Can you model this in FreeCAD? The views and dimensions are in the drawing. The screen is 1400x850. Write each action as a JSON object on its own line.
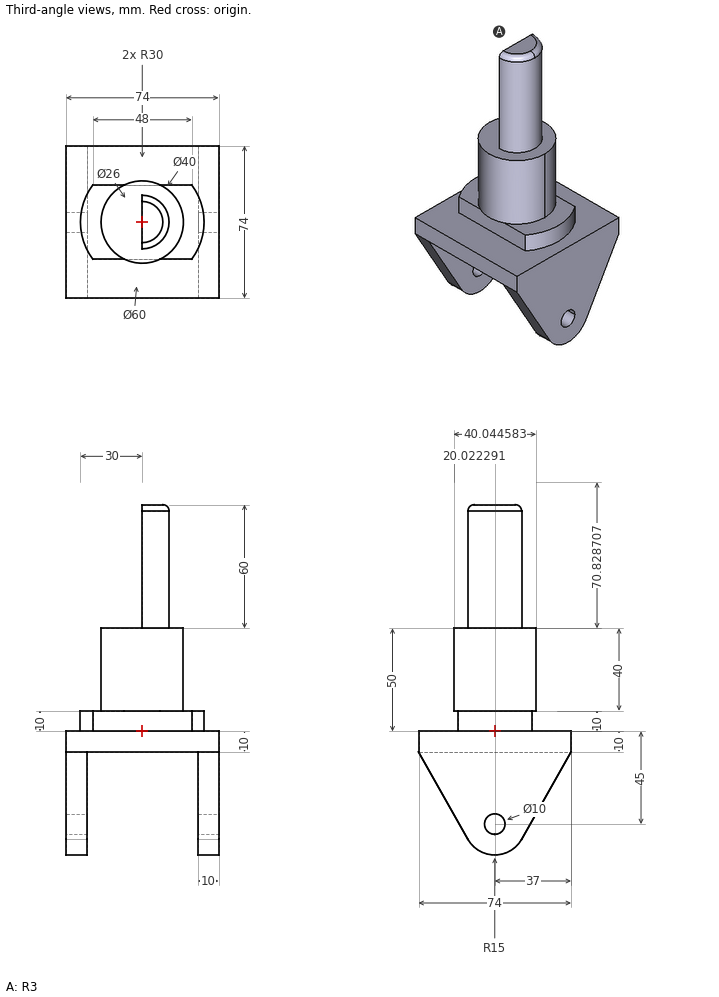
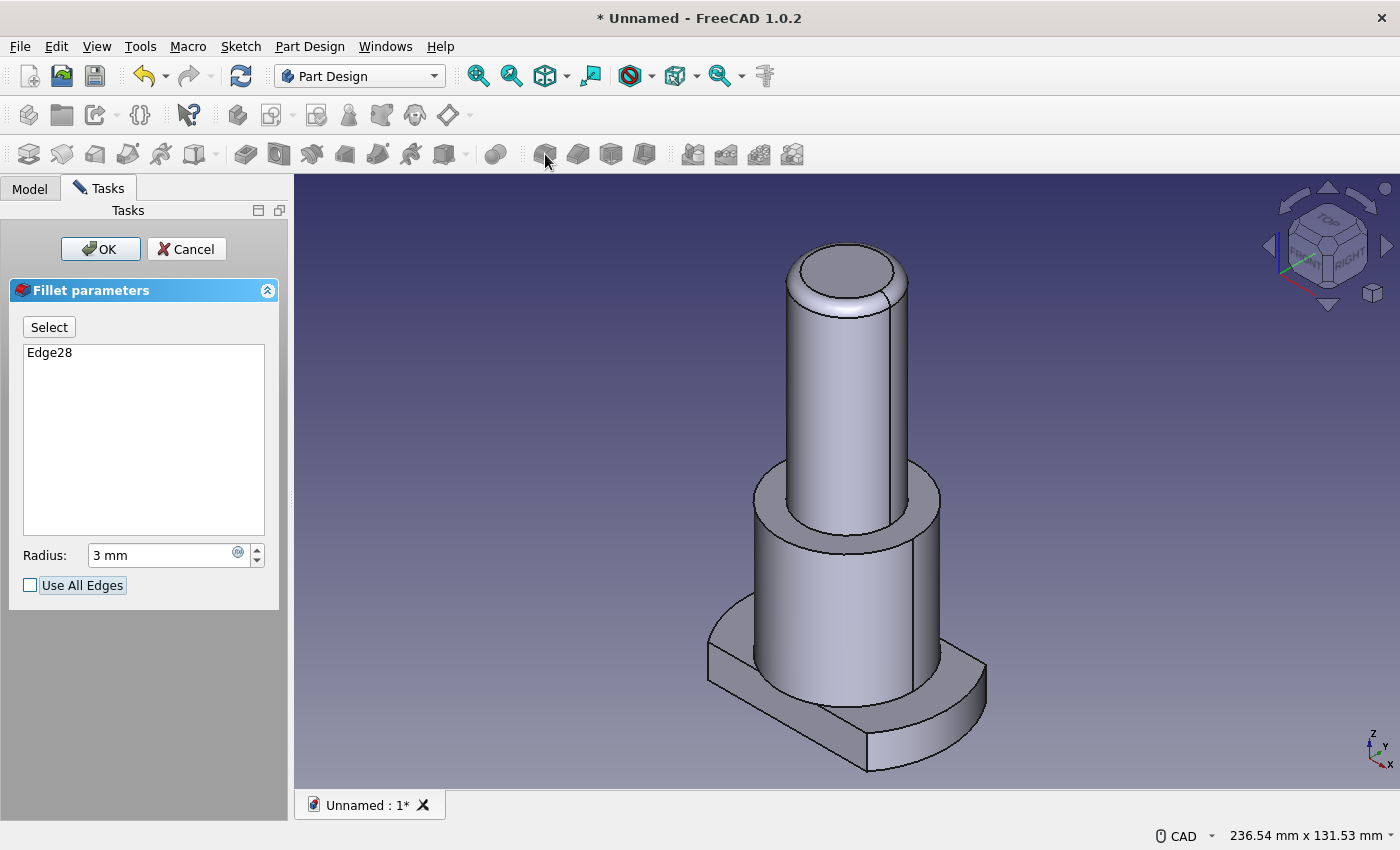
{"action": "left_click", "coordinate": [101, 249]}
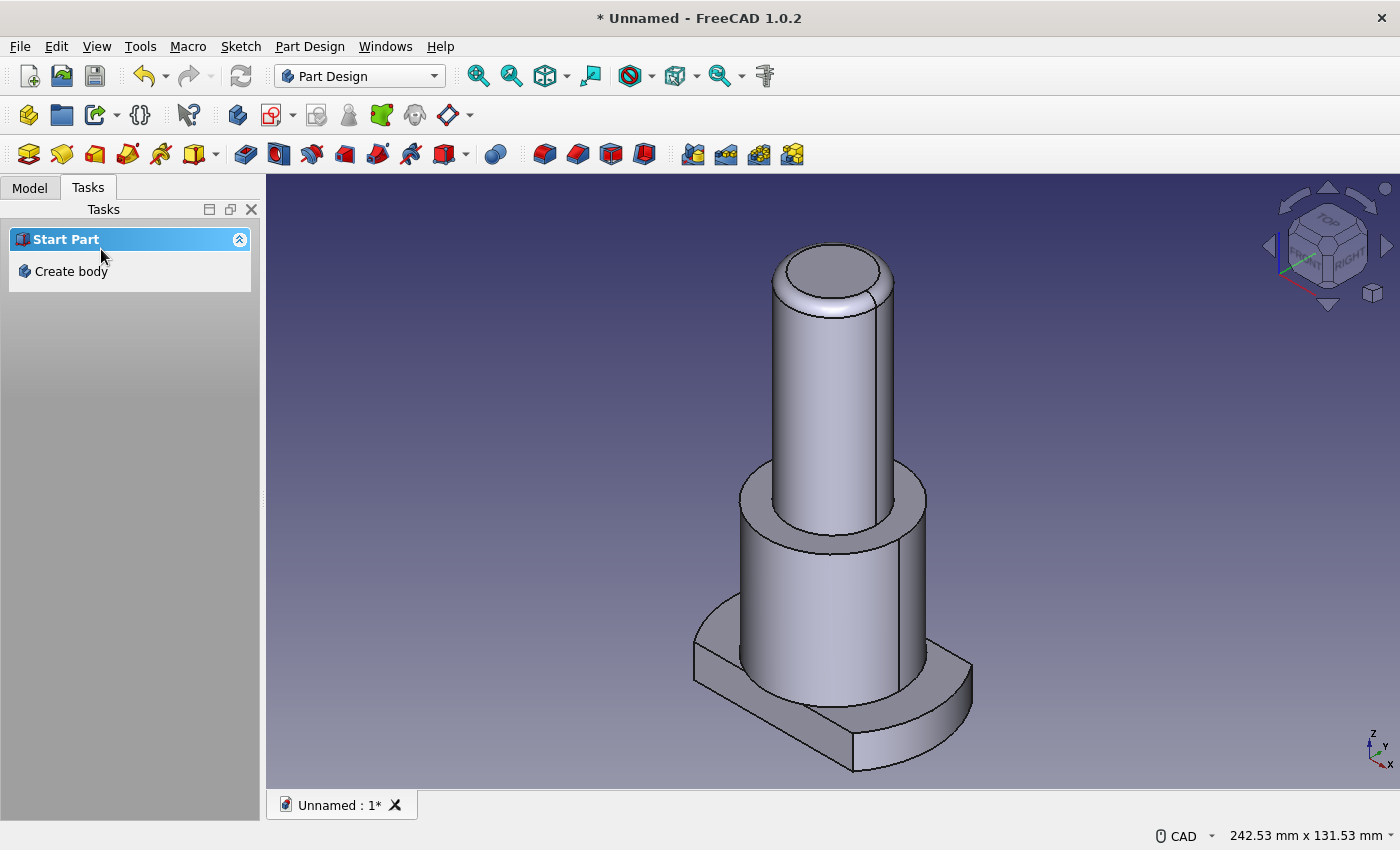
{"action": "left_click", "coordinate": [270, 116]}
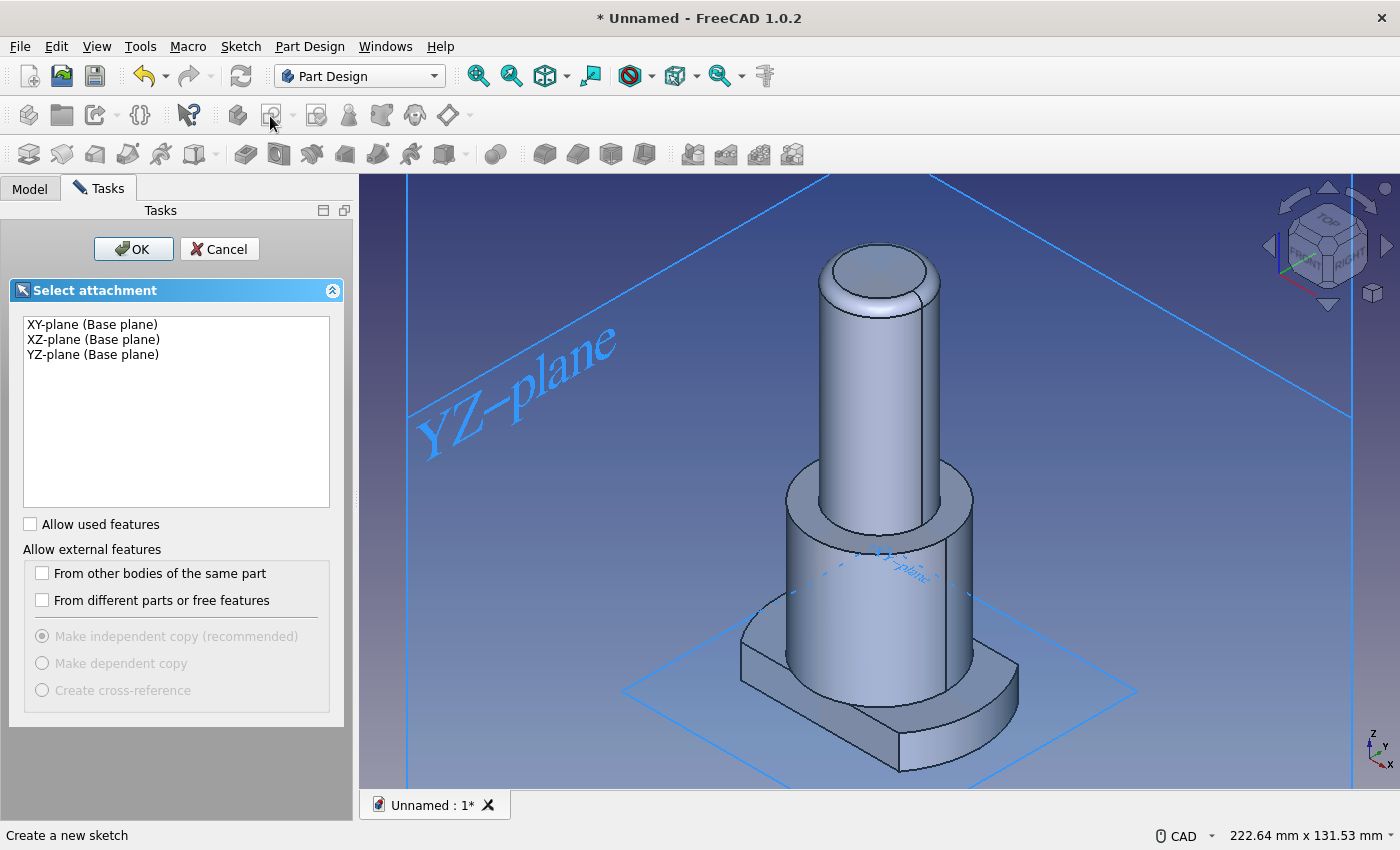
{"action": "left_click", "coordinate": [84, 354]}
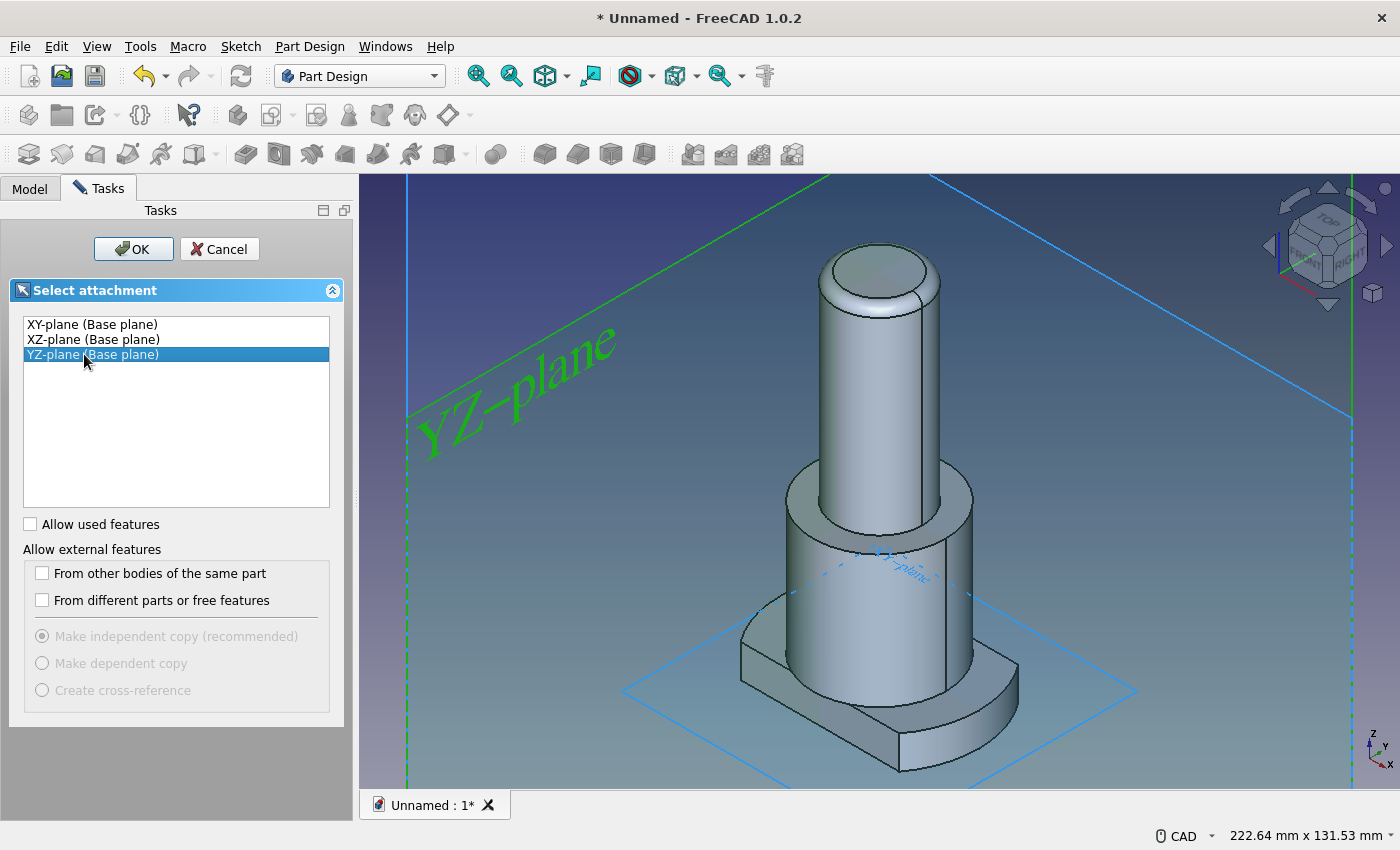
{"action": "left_click", "coordinate": [134, 249]}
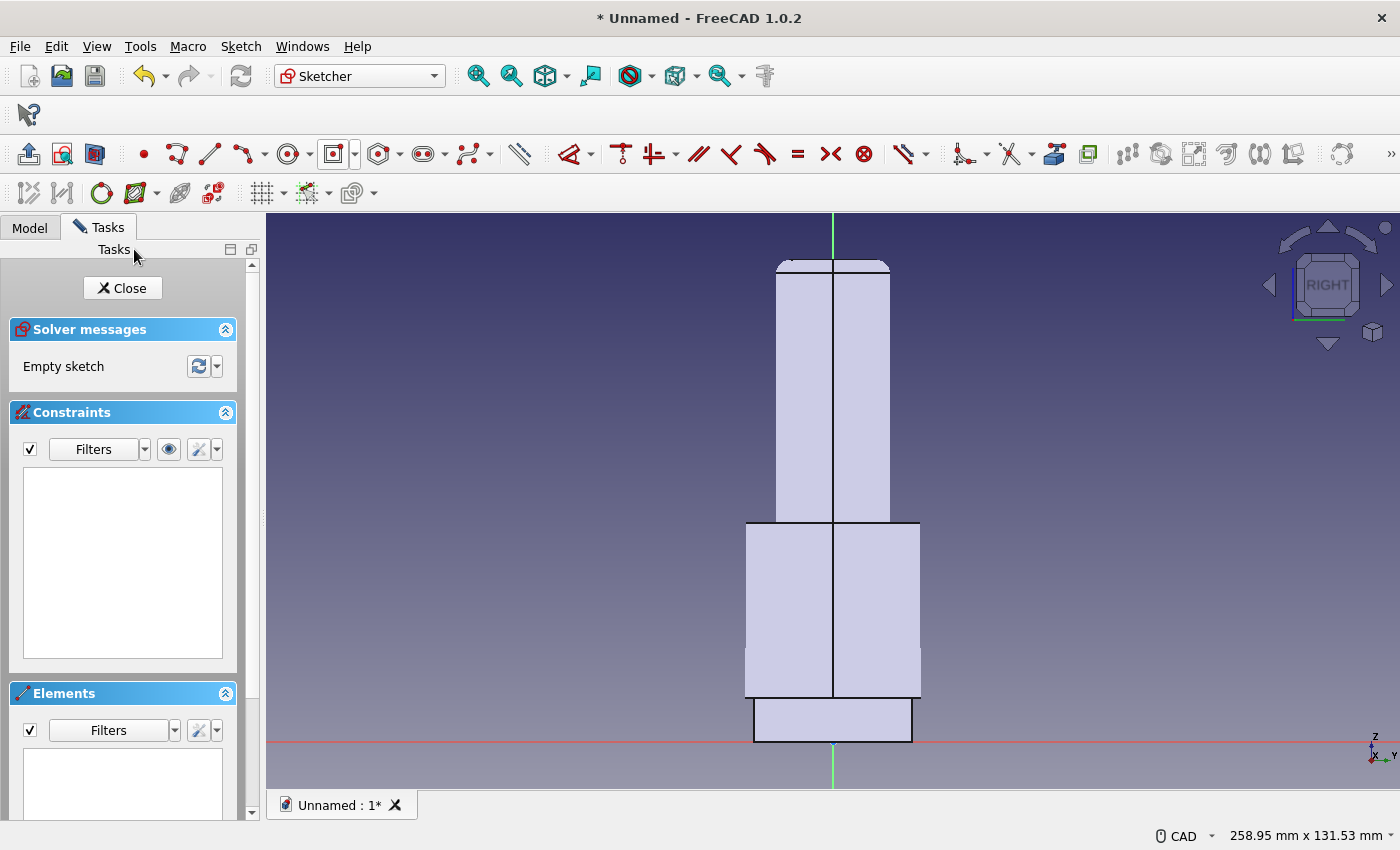
{"action": "left_click", "coordinate": [95, 154]}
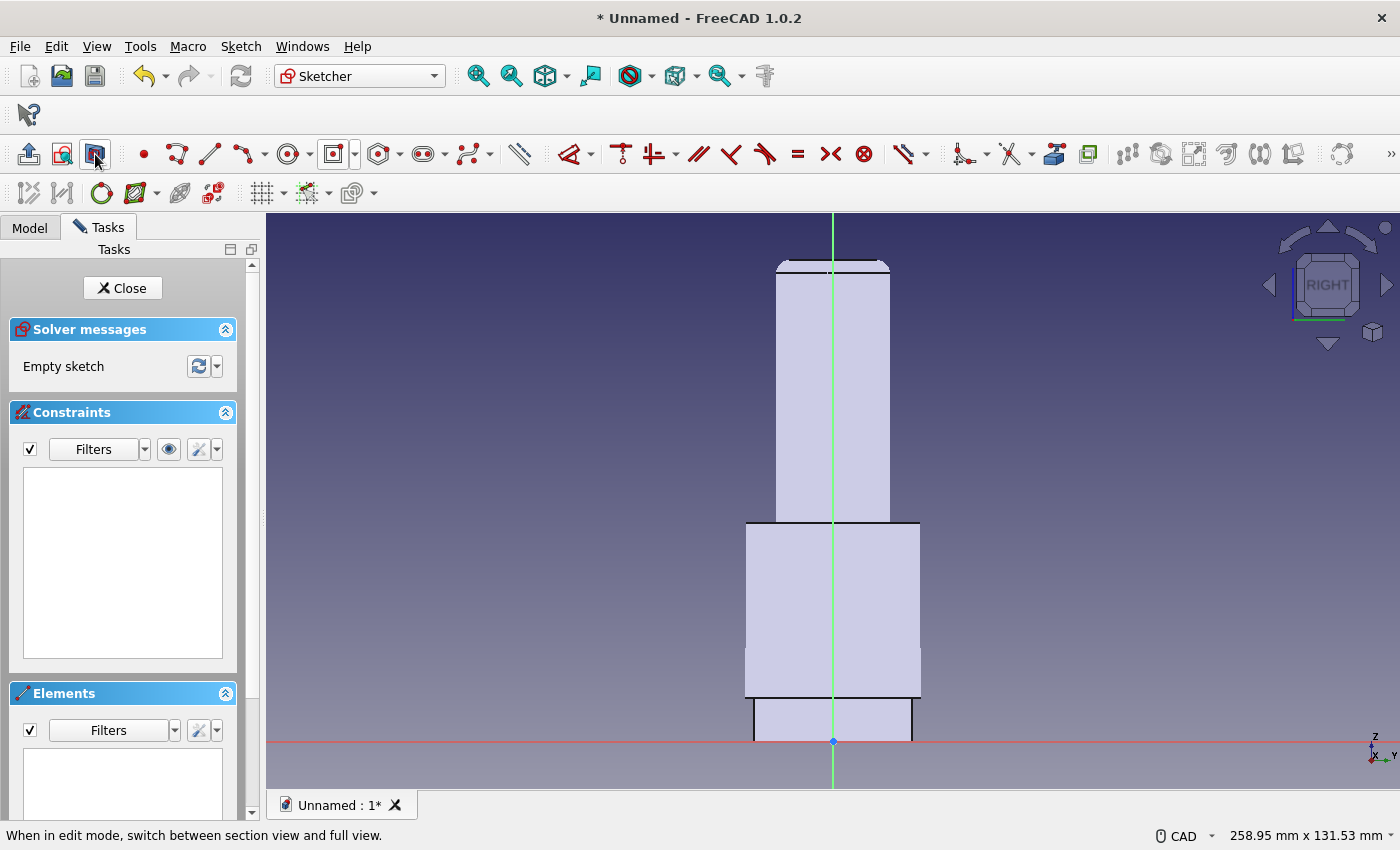
{"action": "scroll", "coordinate": [625, 549], "scroll_direction": "down", "scroll_amount": 2}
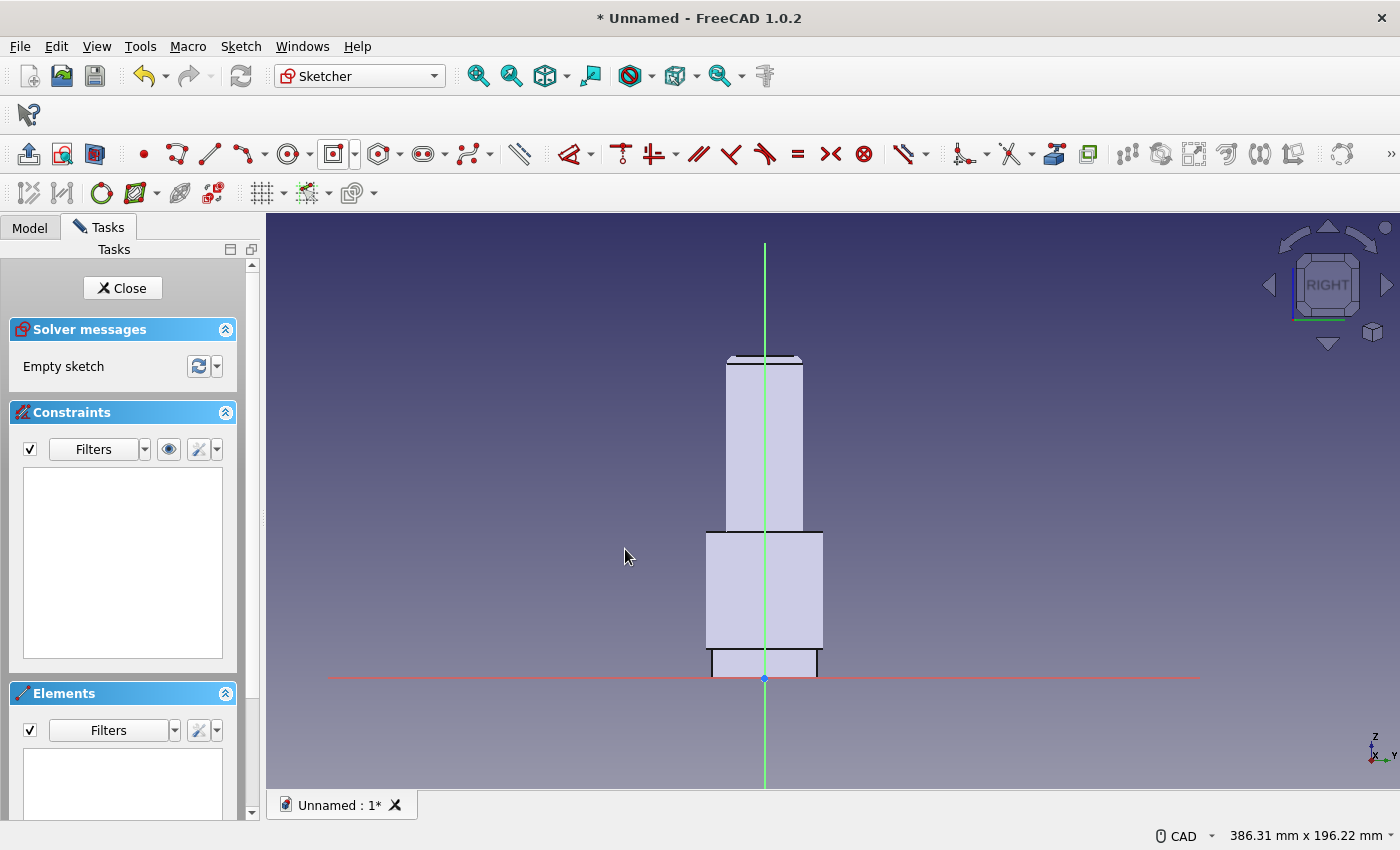
{"action": "key", "text": "g r"}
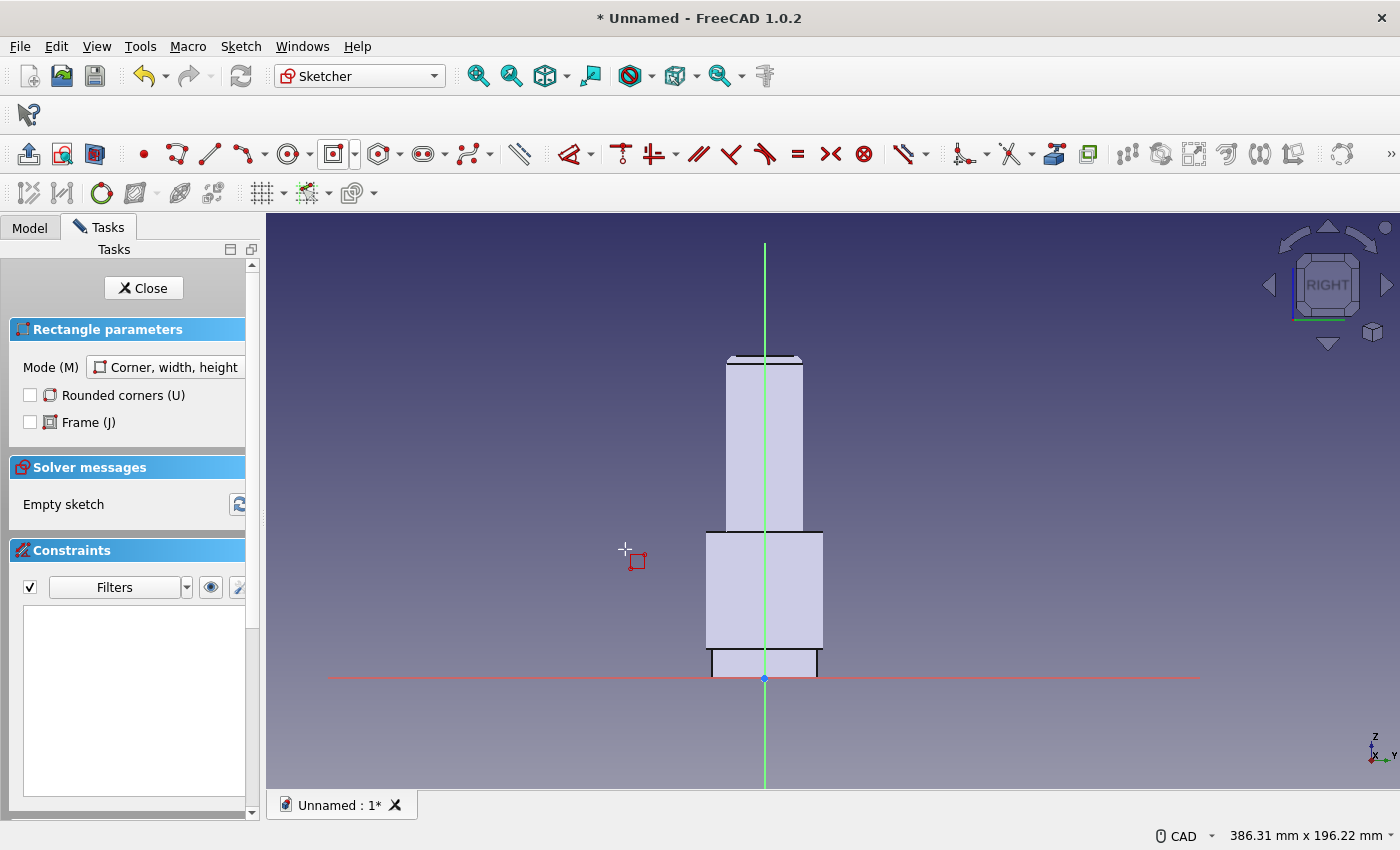
{"action": "left_click", "coordinate": [706, 324]}
{"action": "mouse_move", "coordinate": [823, 532]}